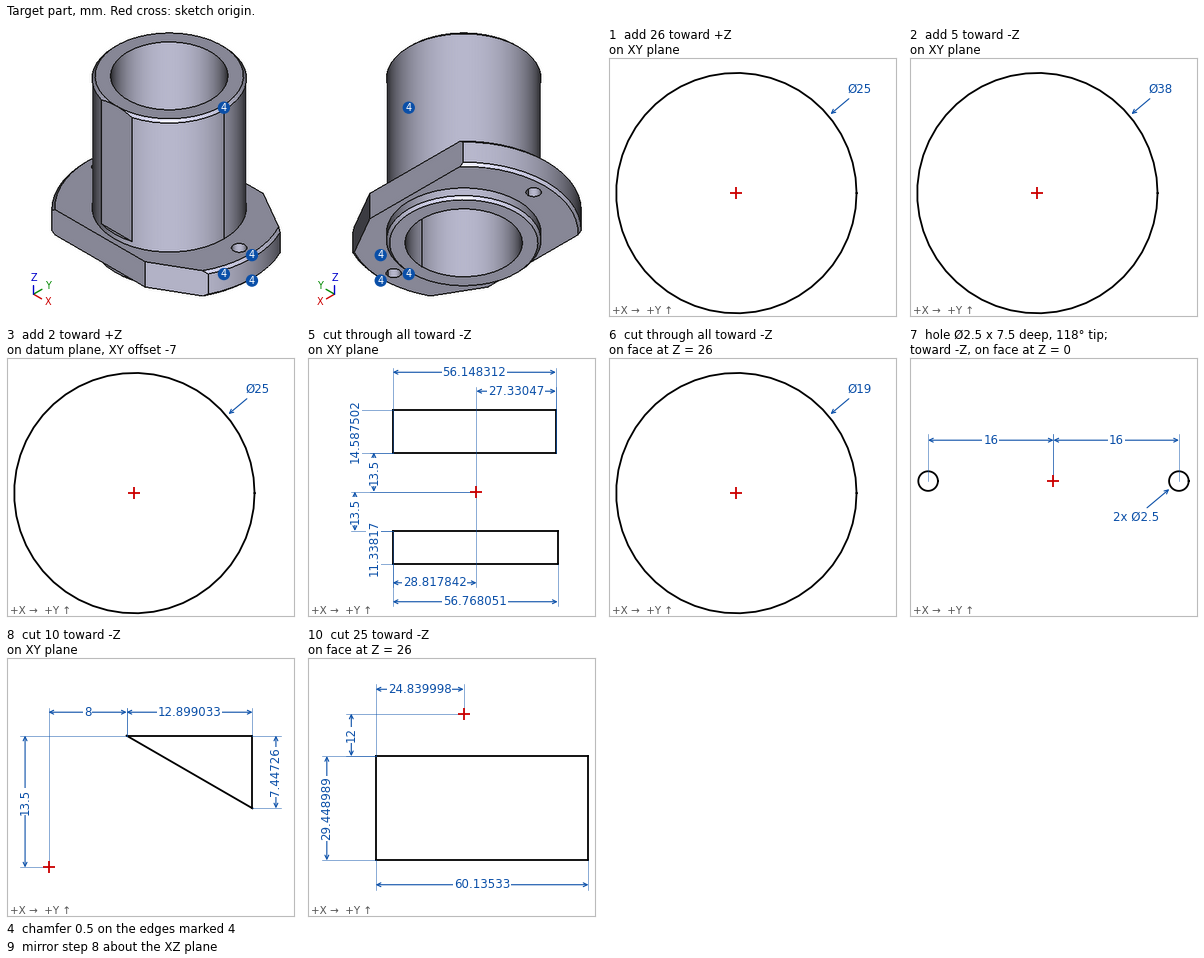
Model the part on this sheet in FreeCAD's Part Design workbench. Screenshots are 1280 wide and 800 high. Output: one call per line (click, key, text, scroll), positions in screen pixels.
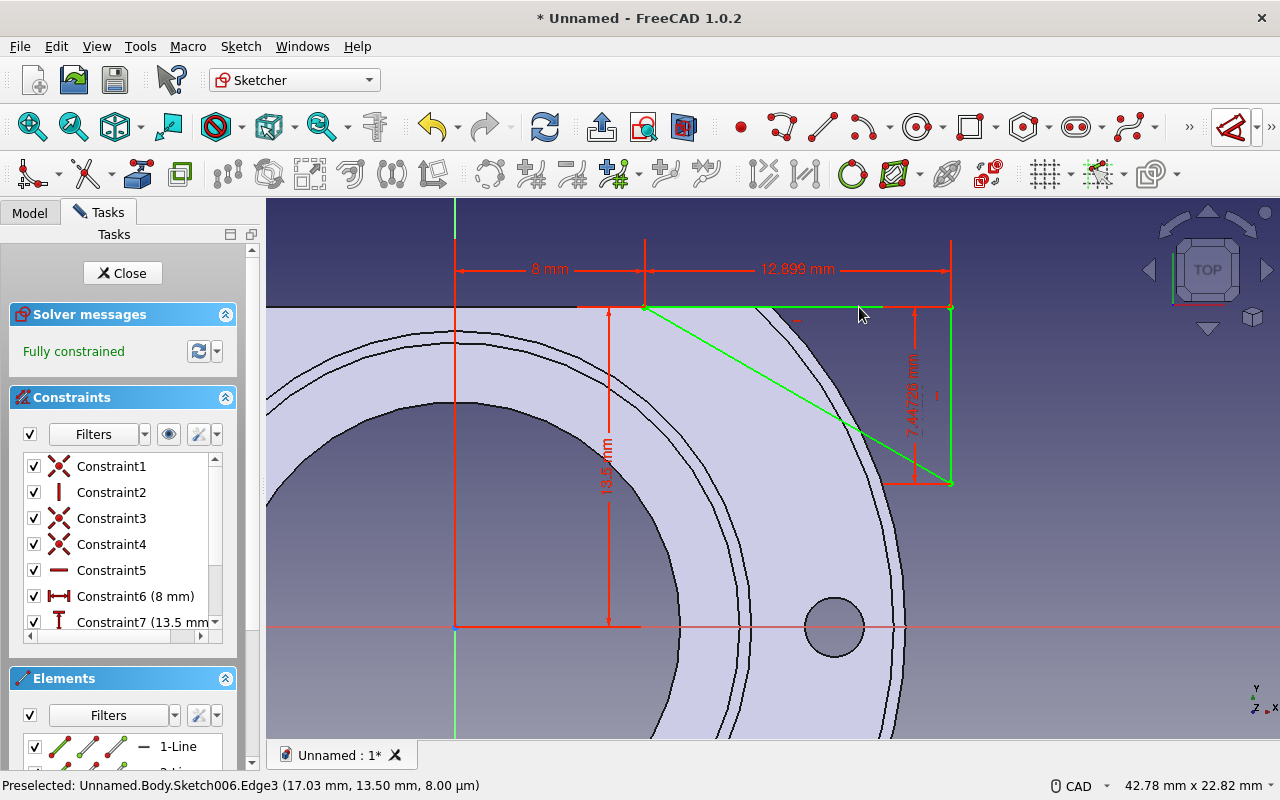
click(123, 273)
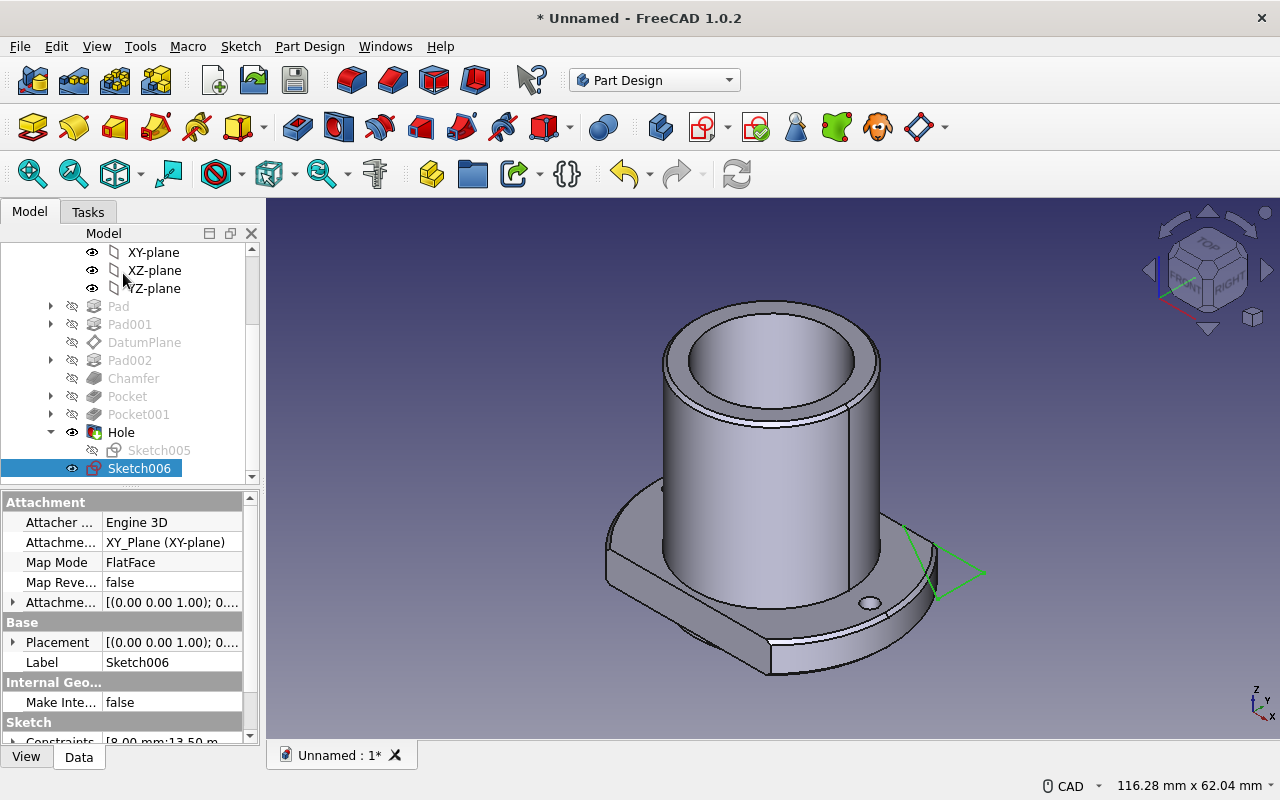
click(298, 128)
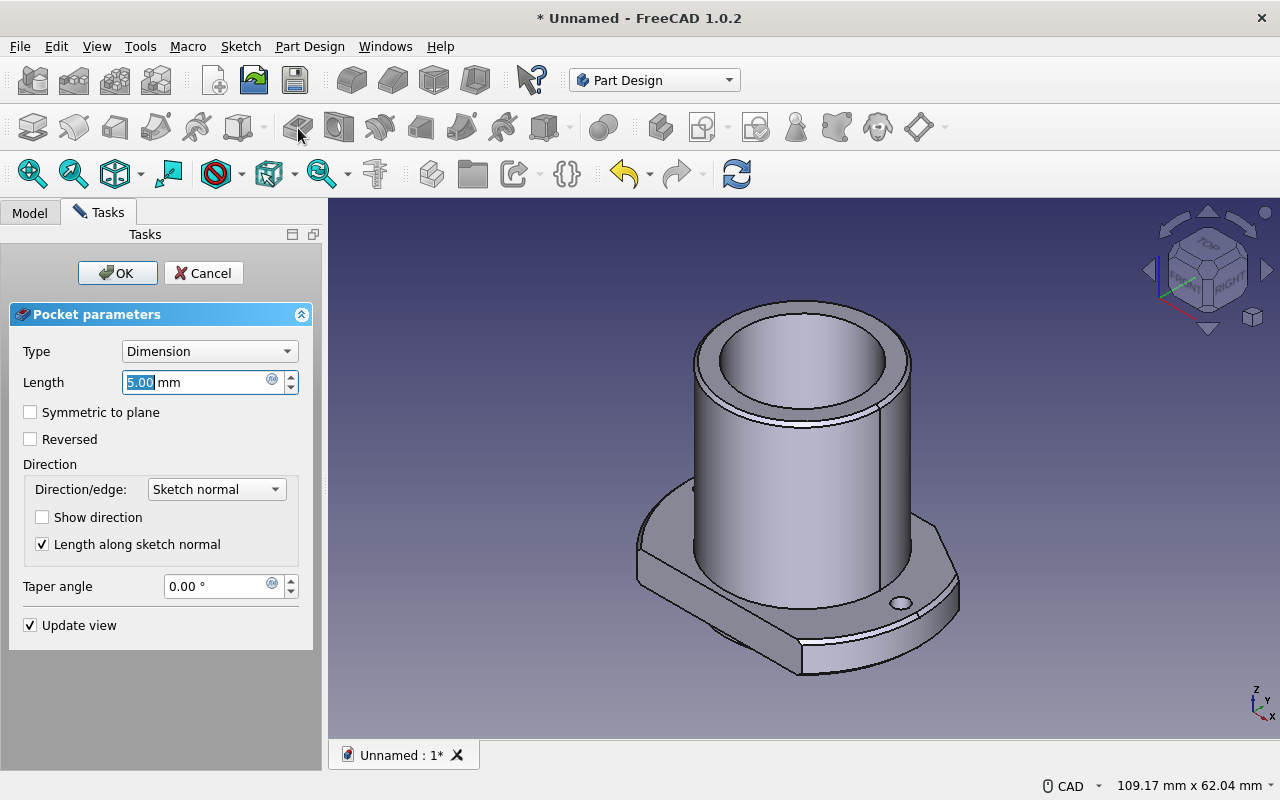
text(10)
key(Tab)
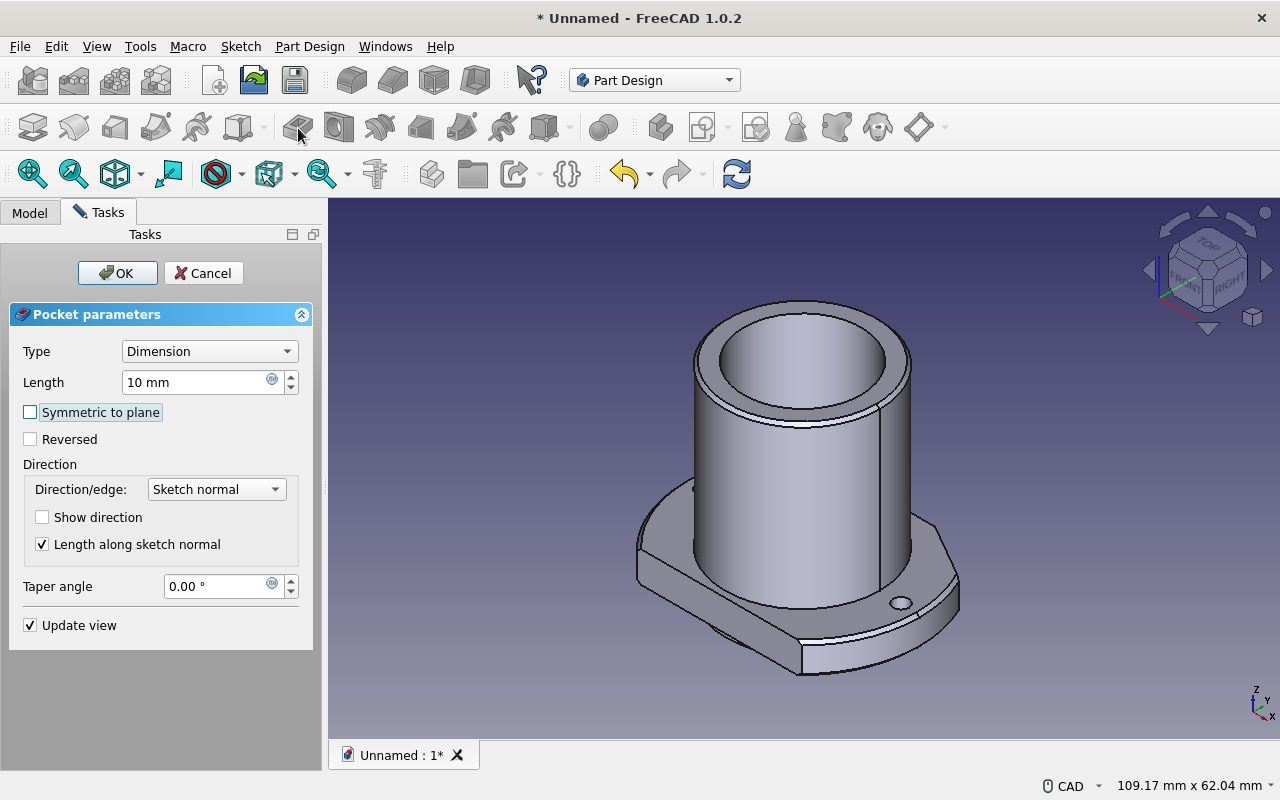
click(118, 273)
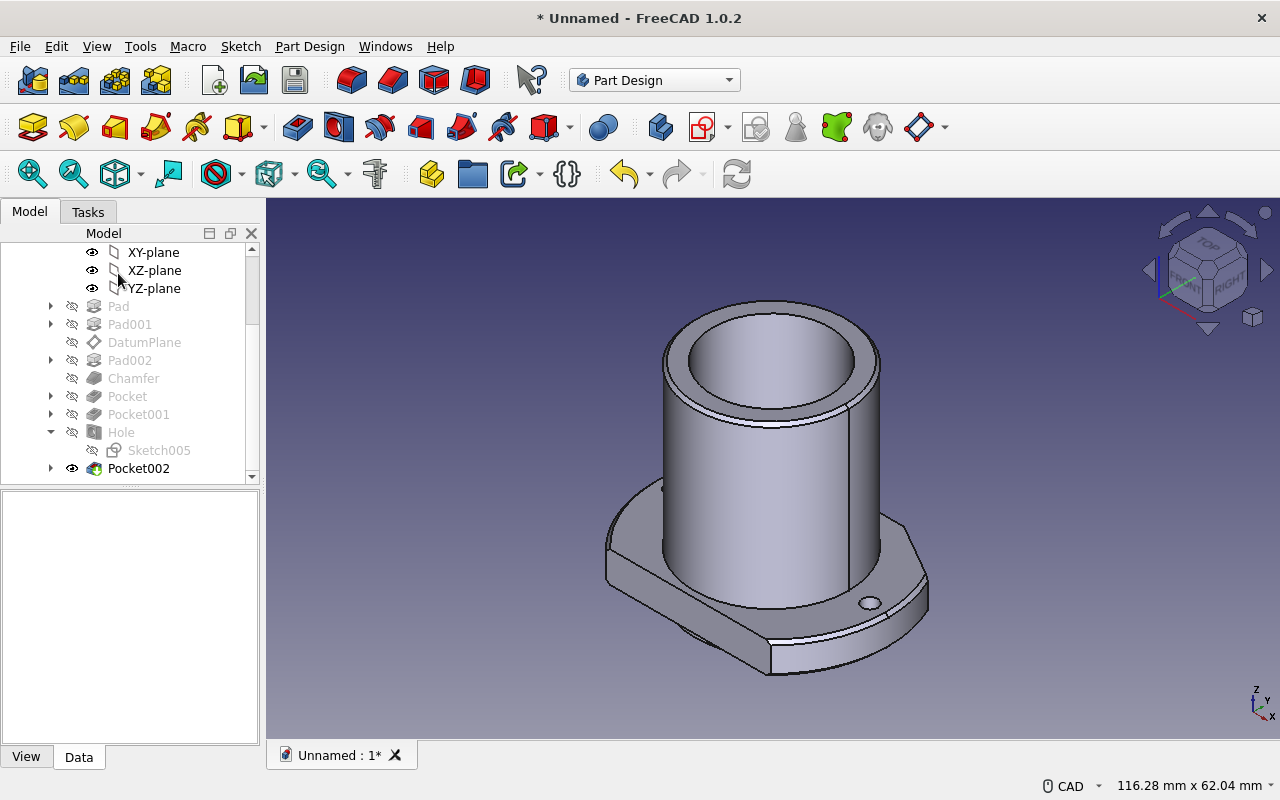
click(117, 468)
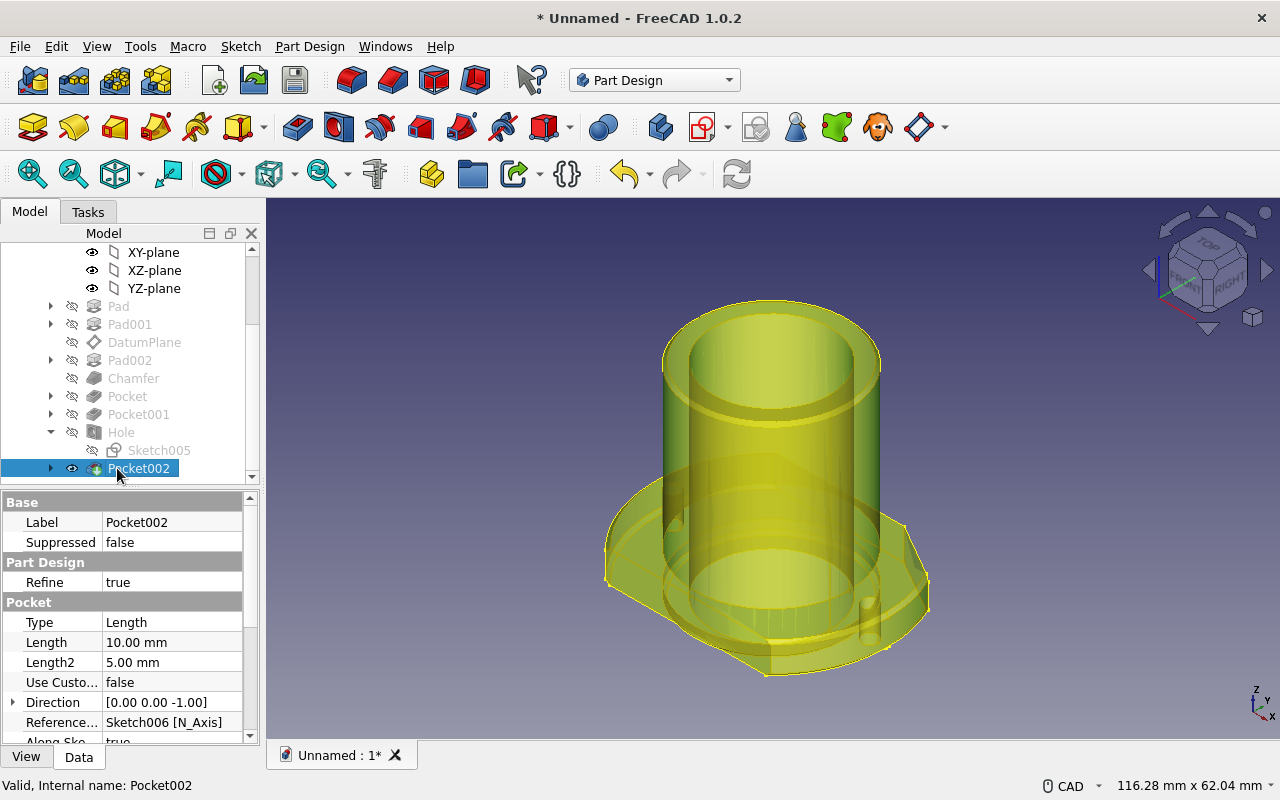
click(33, 80)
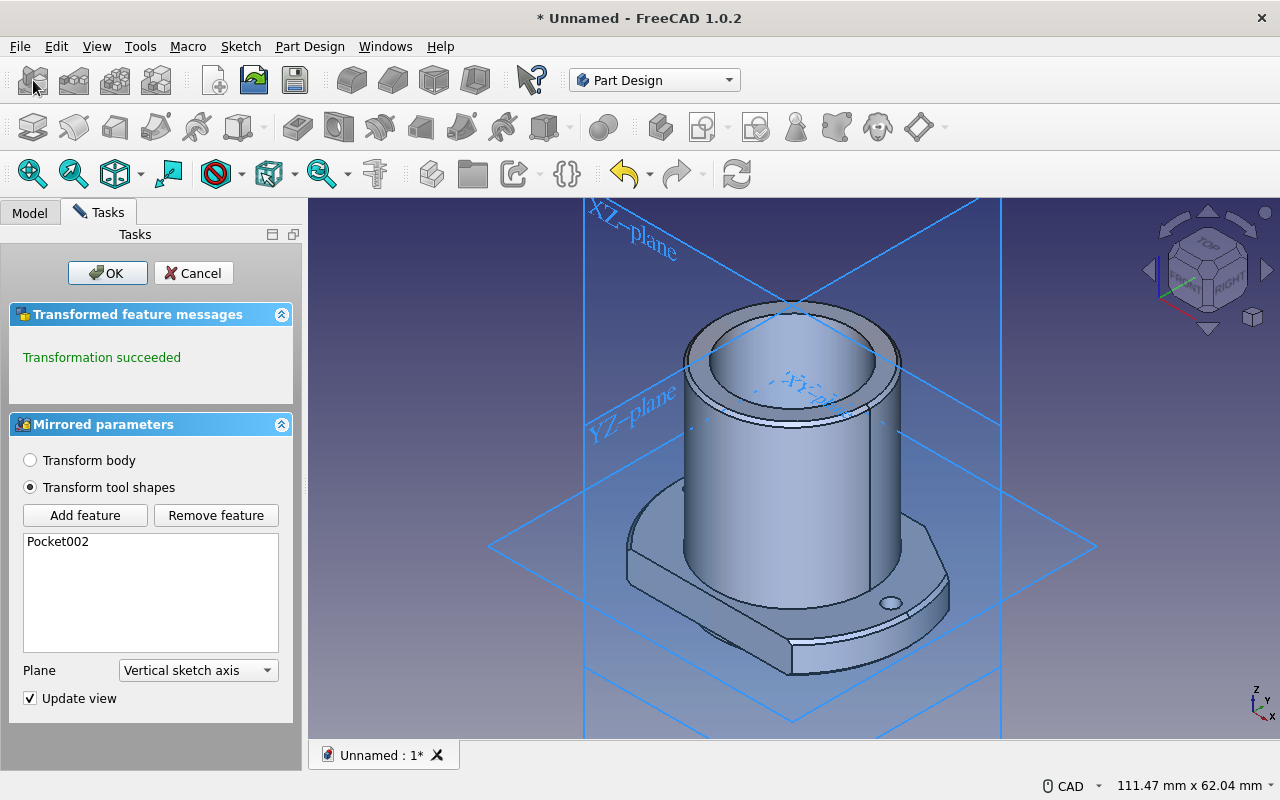
click(199, 670)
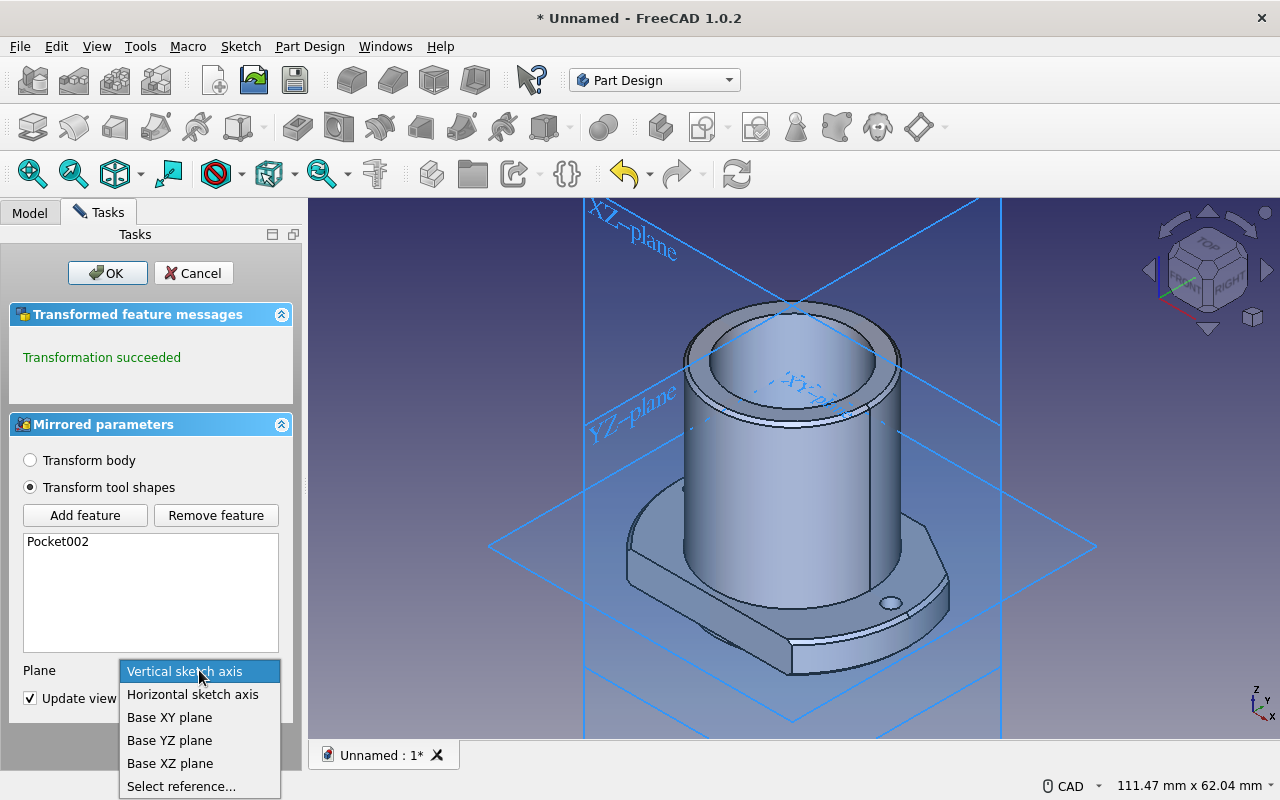
click(198, 764)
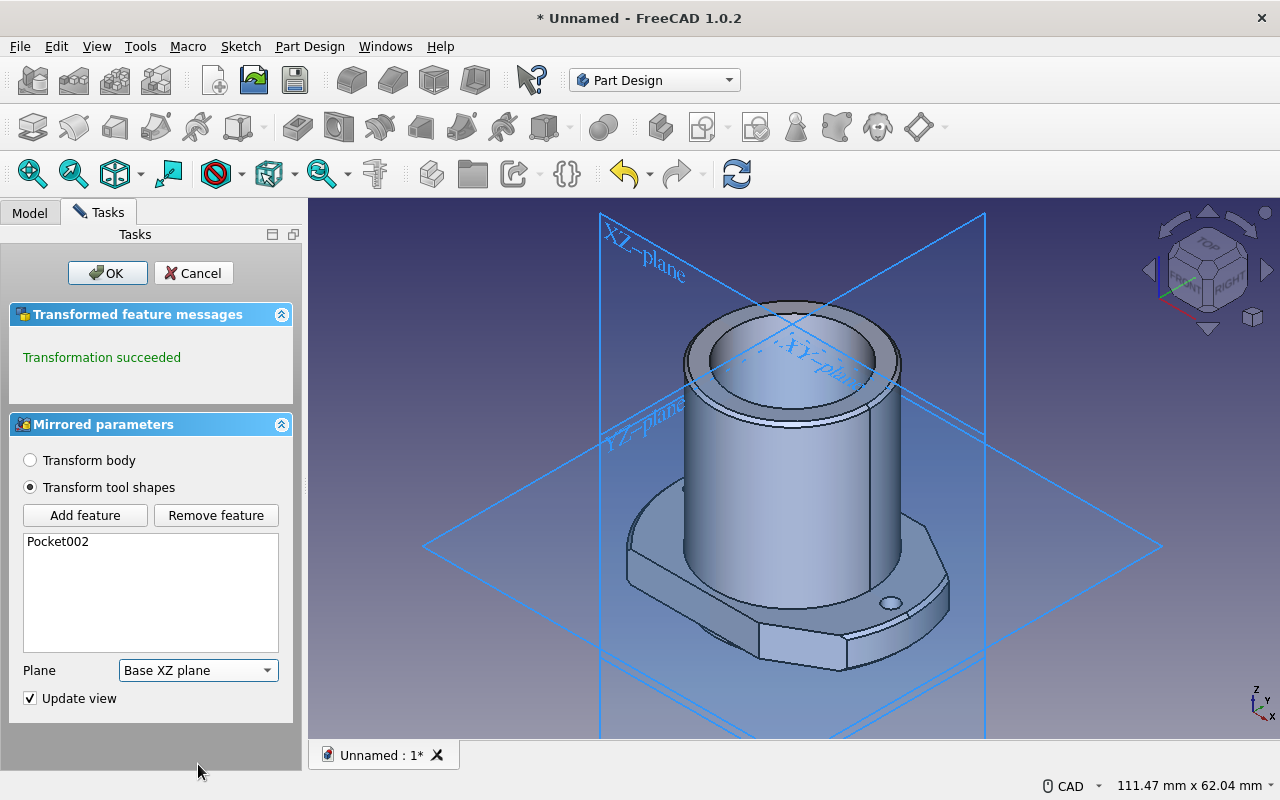
click(108, 273)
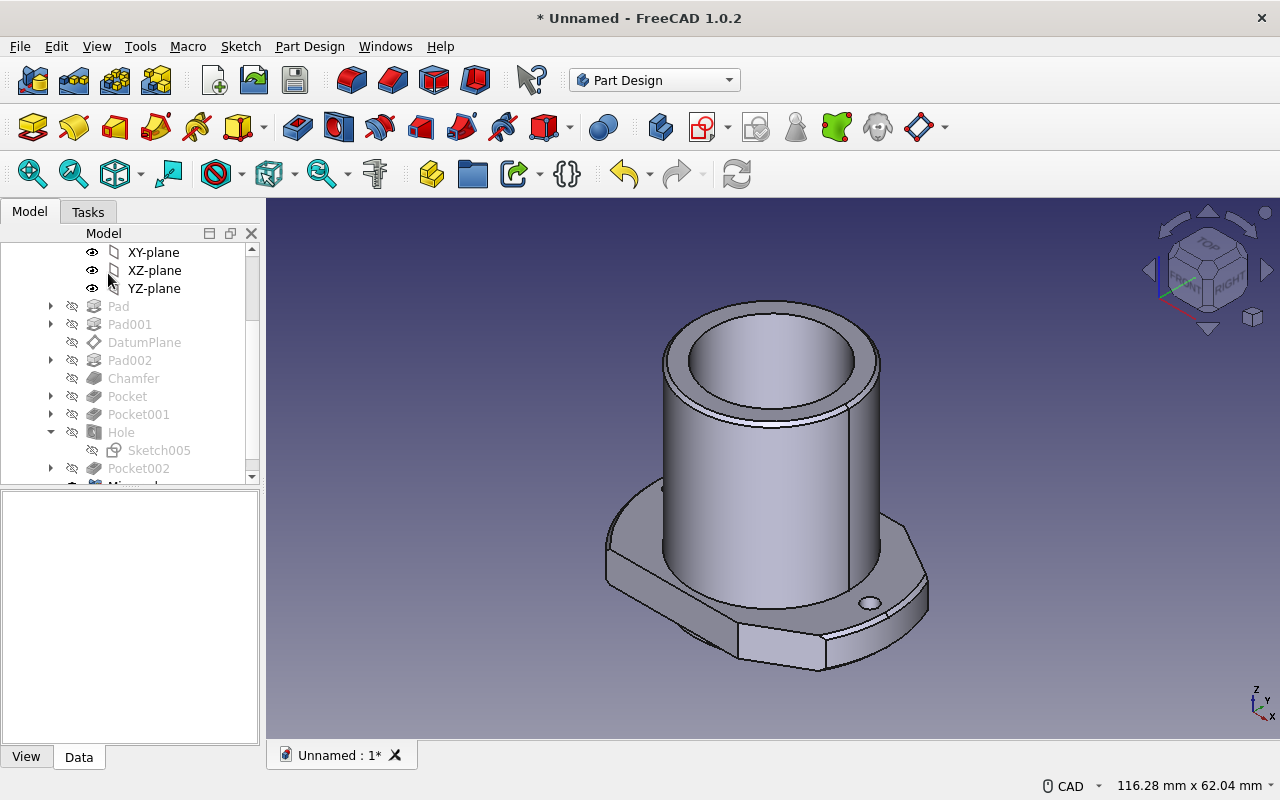
click(856, 336)